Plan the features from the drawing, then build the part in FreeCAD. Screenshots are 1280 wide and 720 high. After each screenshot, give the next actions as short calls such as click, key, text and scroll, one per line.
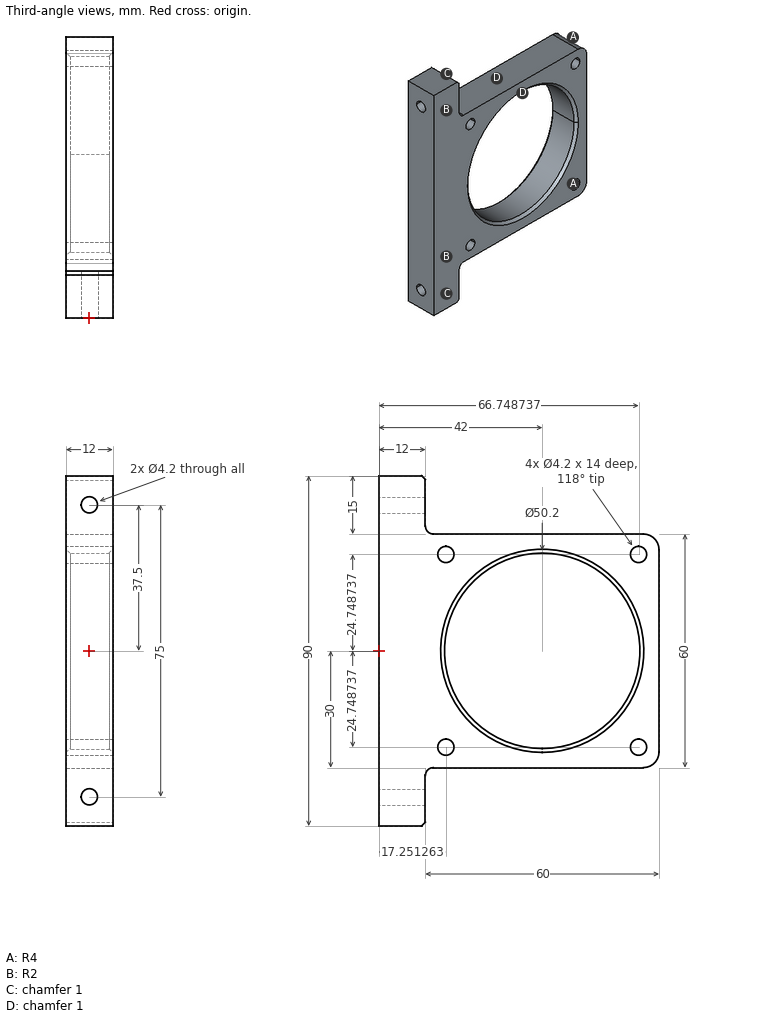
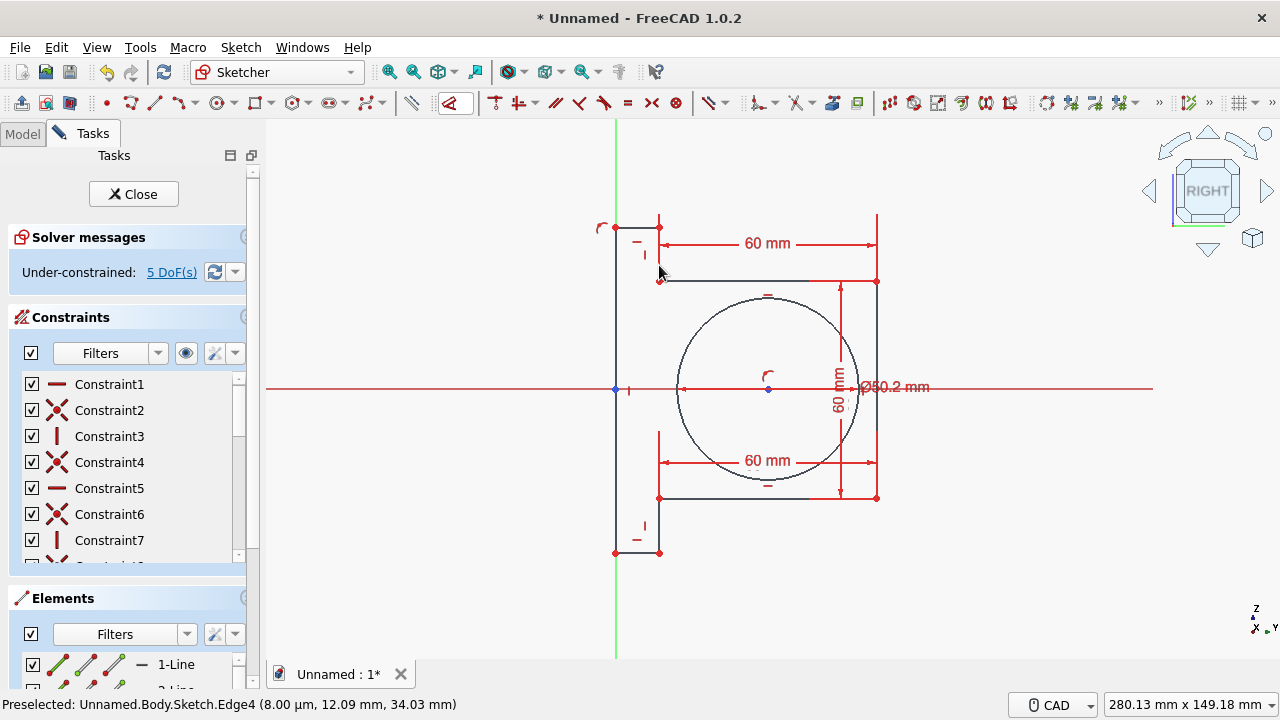
click(468, 104)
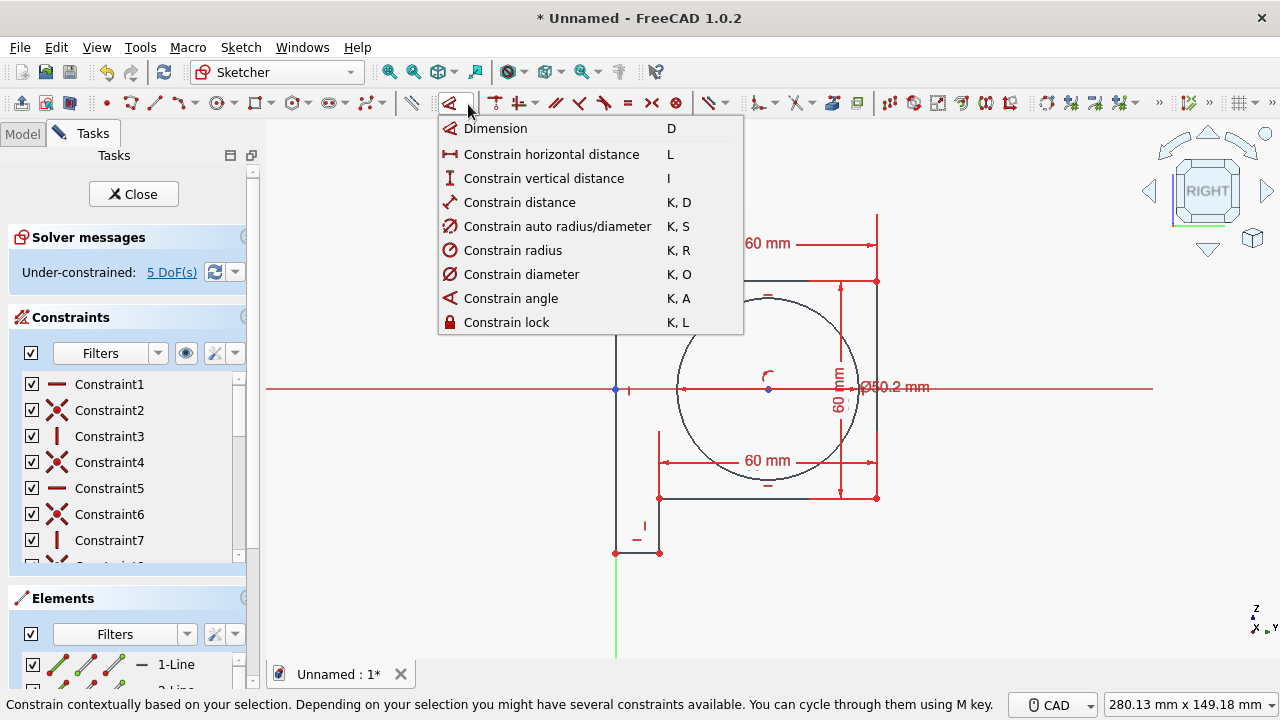
click(591, 178)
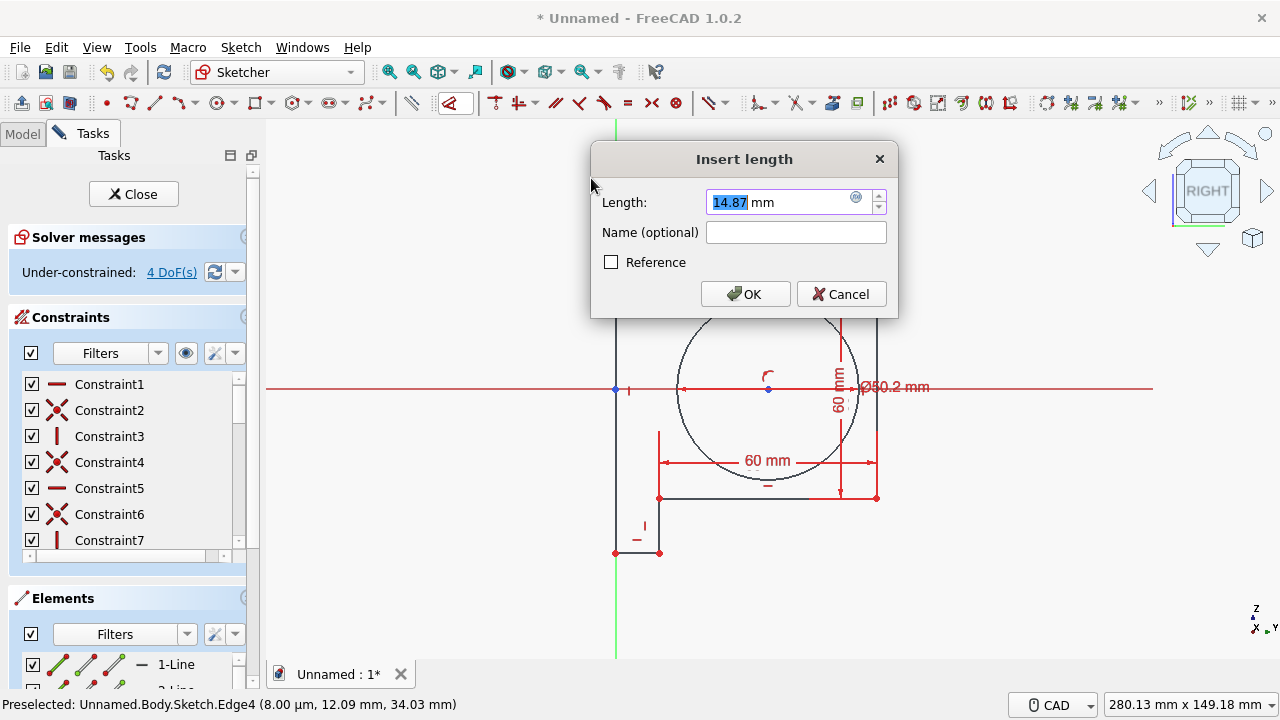
text(15)
key(Return)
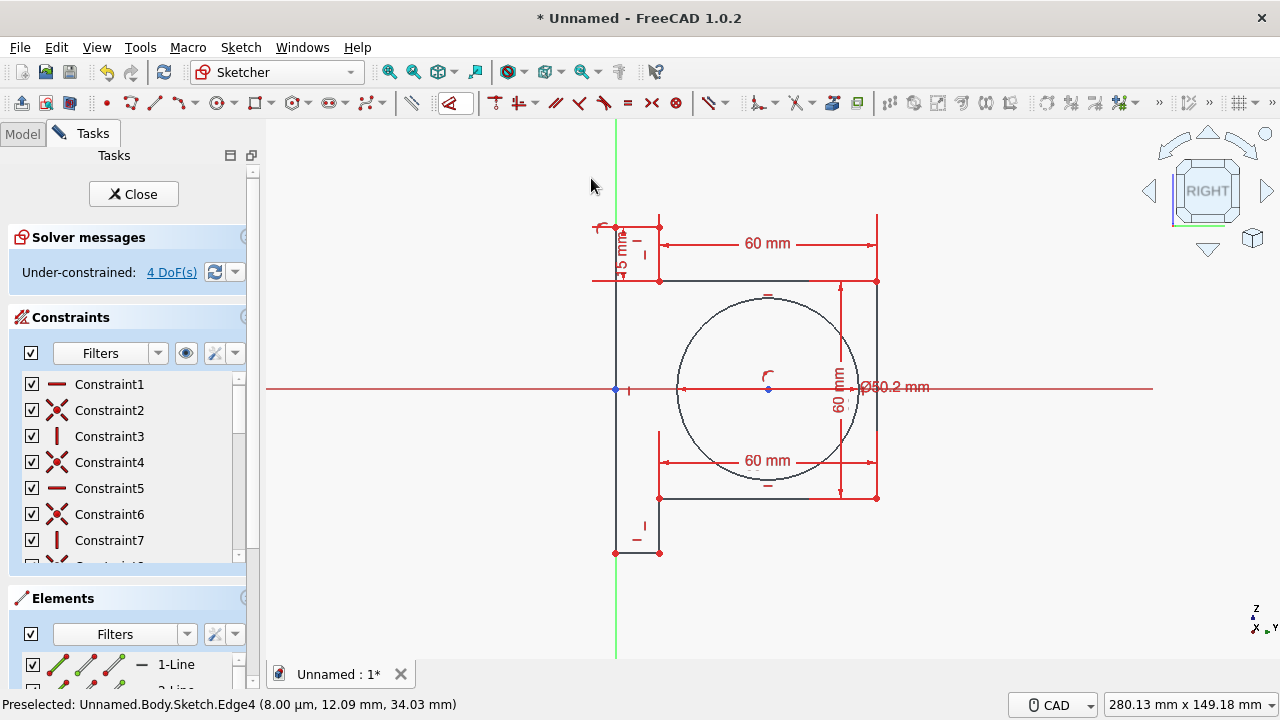
click(646, 227)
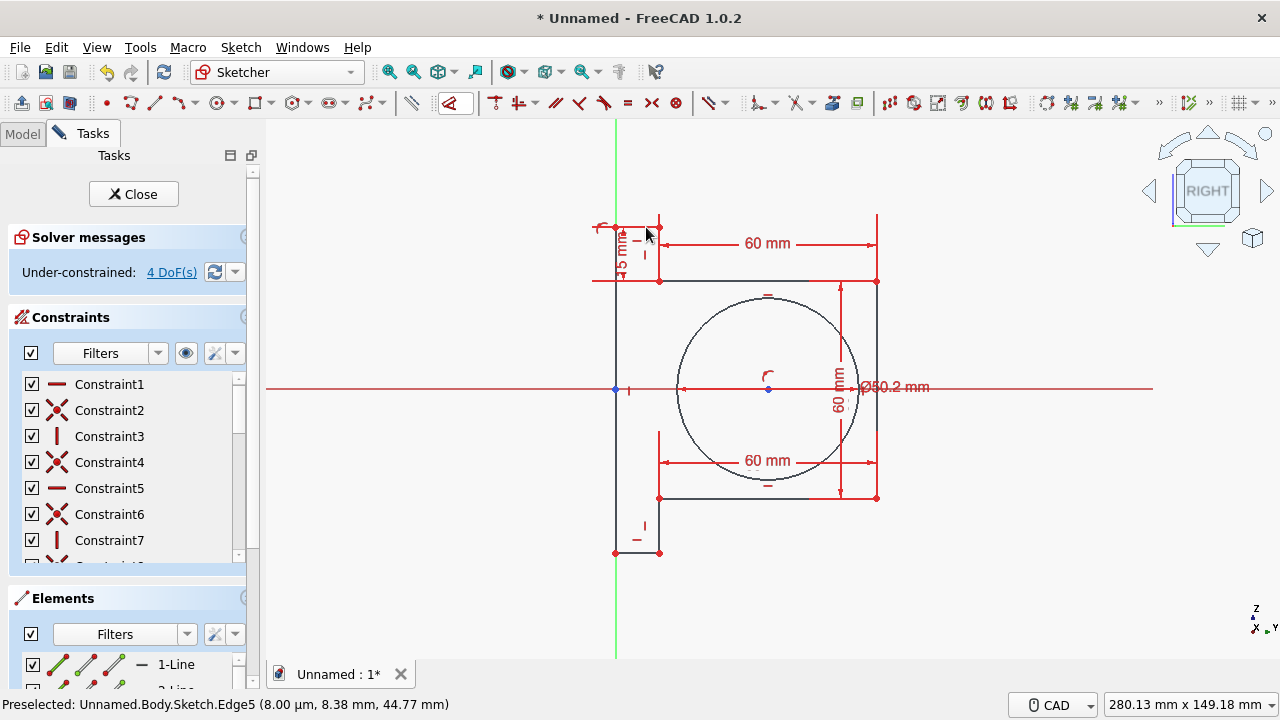
key(l)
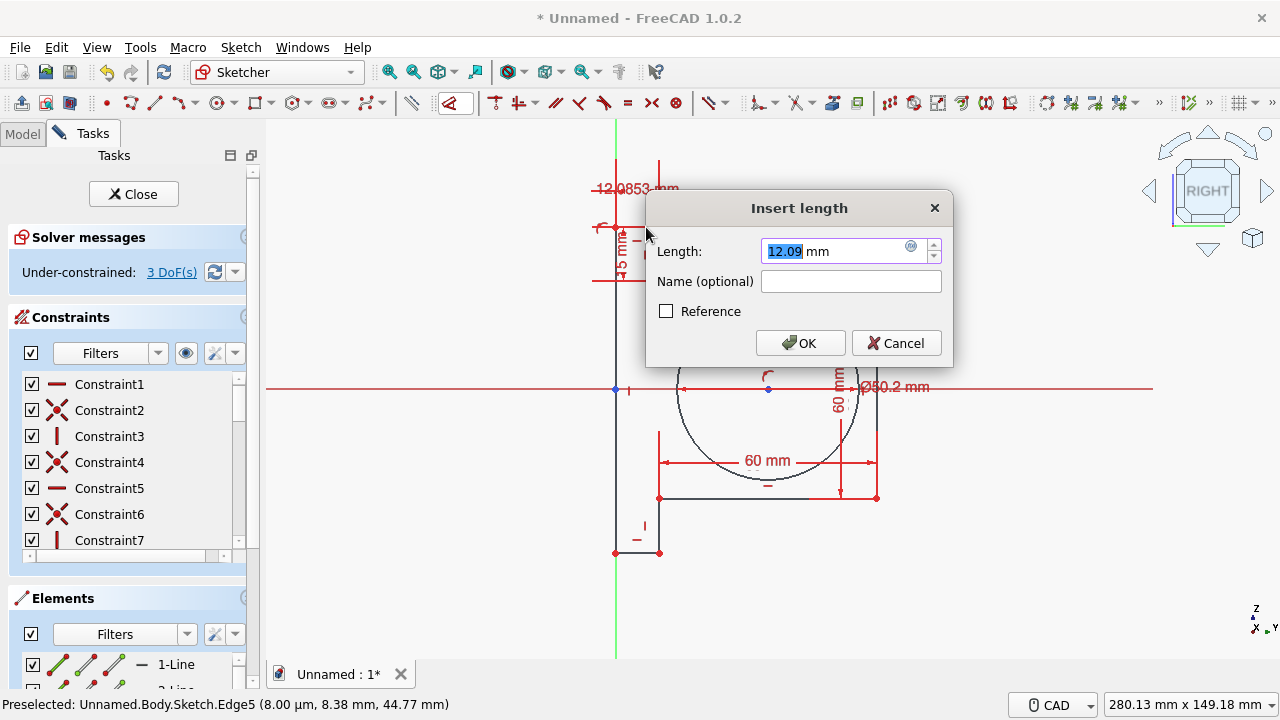
text(12)
key(Return)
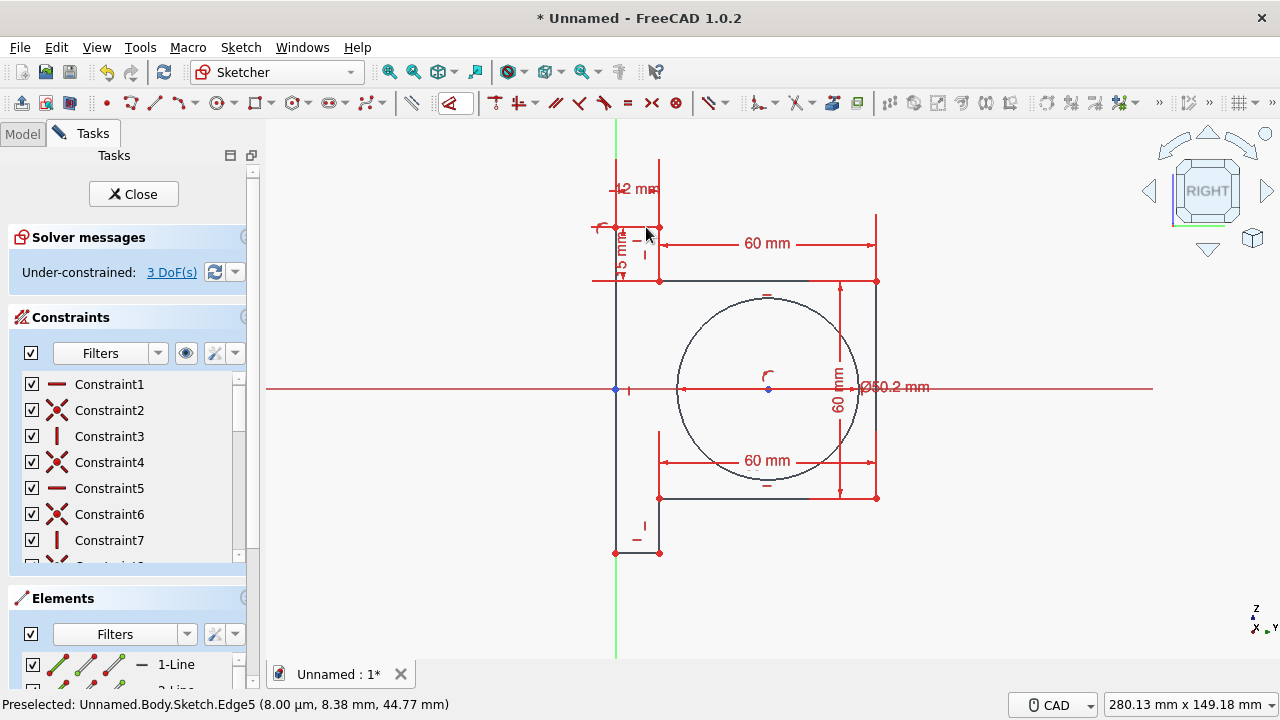
click(616, 325)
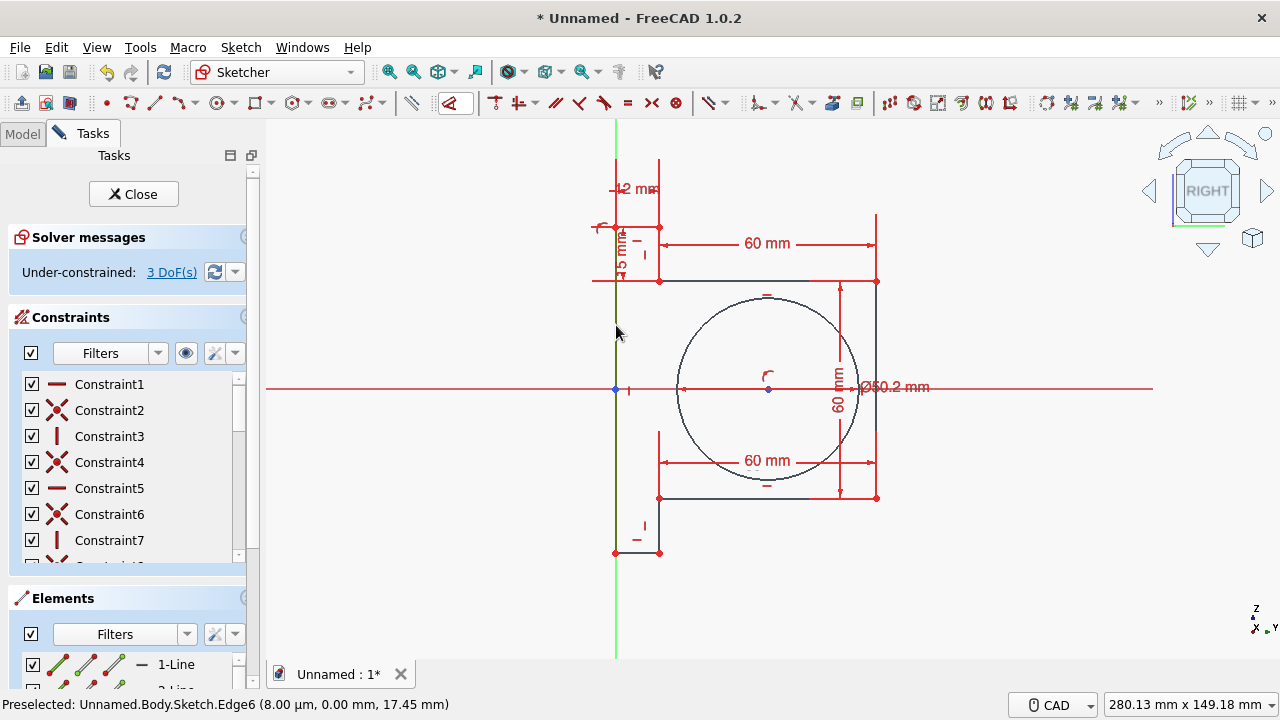
key(i)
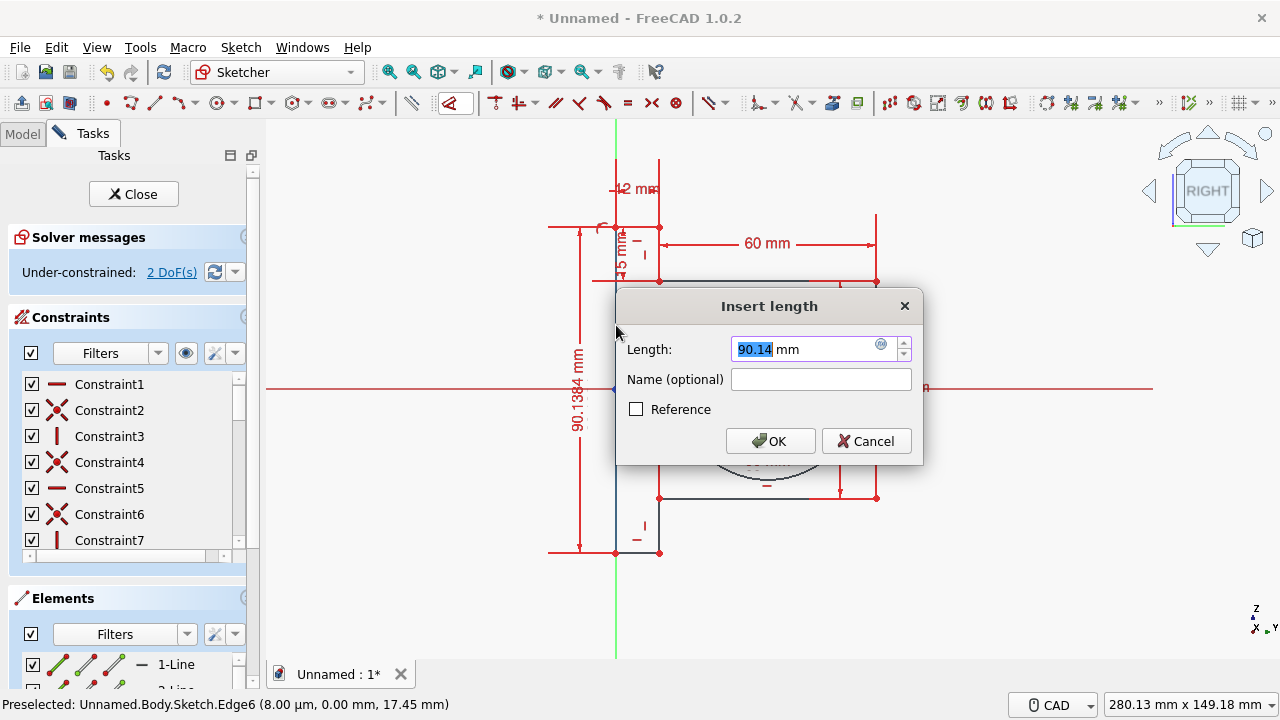
text(90)
key(Return)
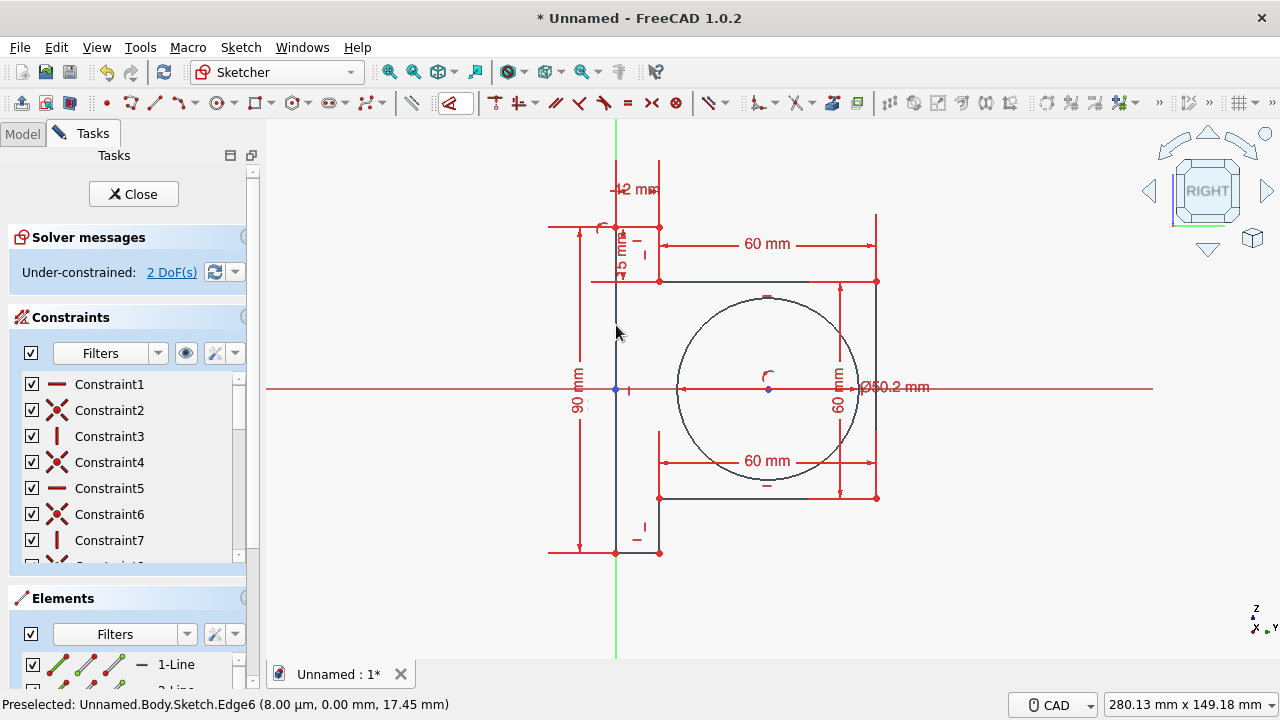
click(768, 389)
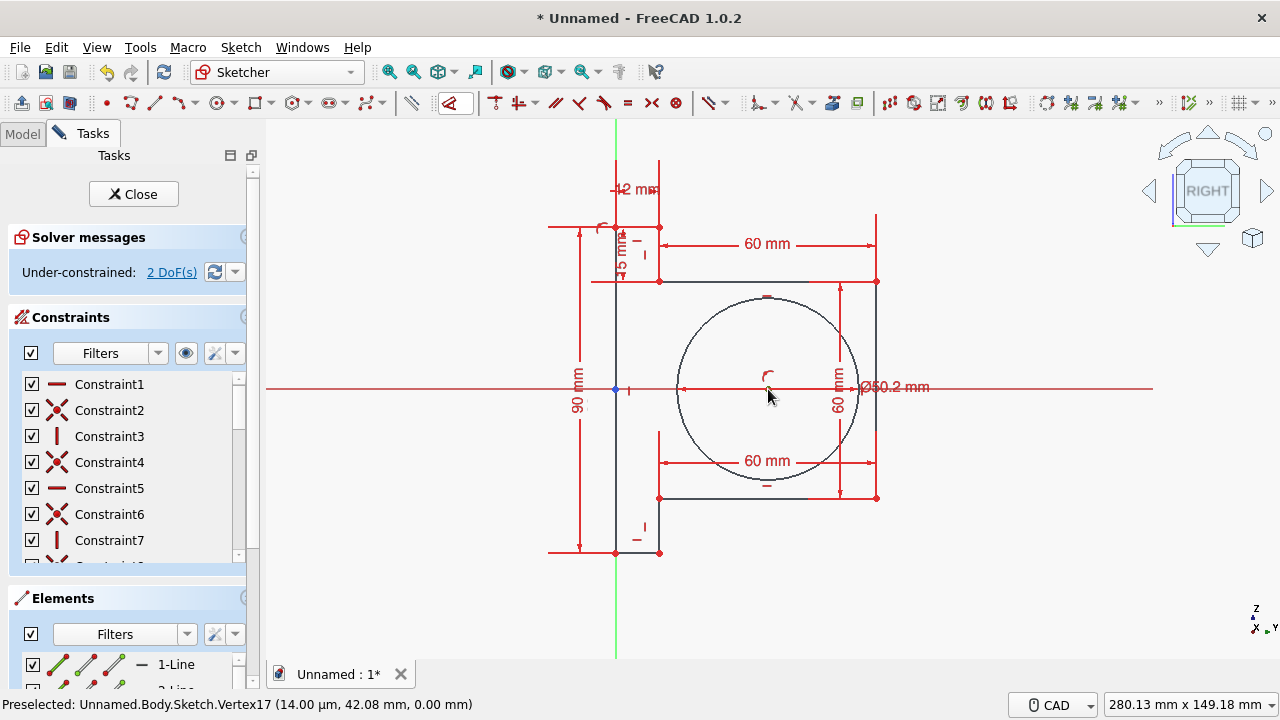
key(l)